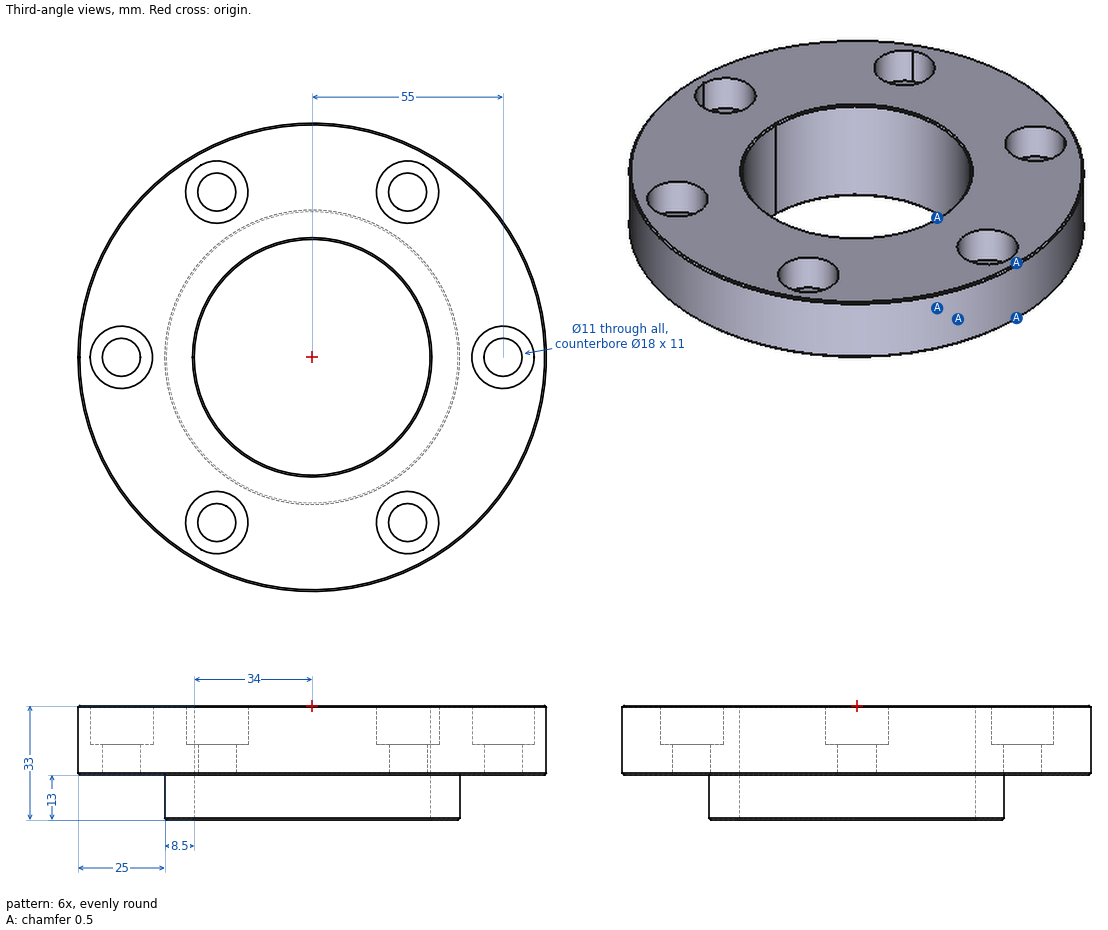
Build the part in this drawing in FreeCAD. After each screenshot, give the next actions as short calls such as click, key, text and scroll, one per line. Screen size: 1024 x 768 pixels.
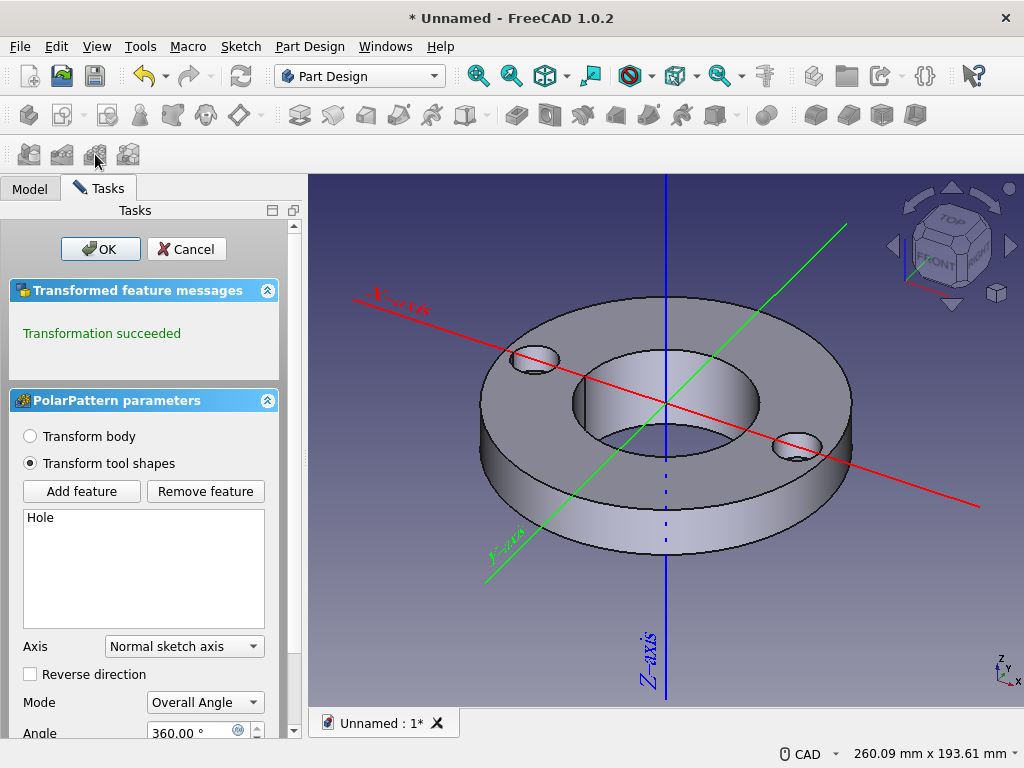
click(185, 646)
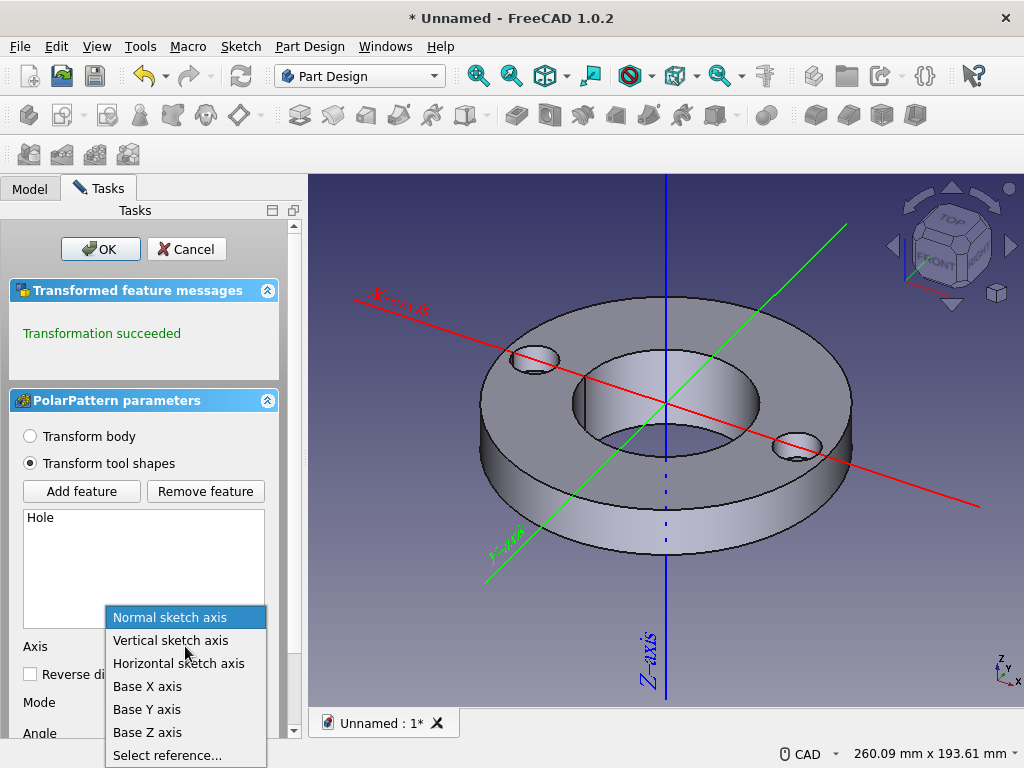
click(184, 732)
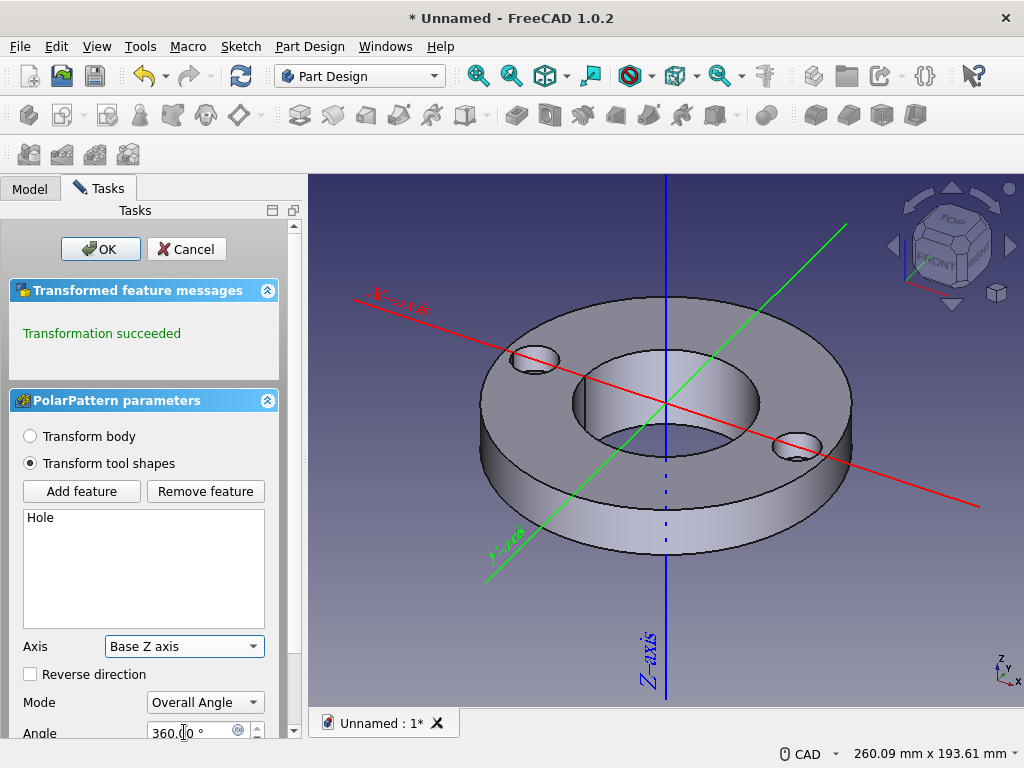
scroll(294, 479, down, 2)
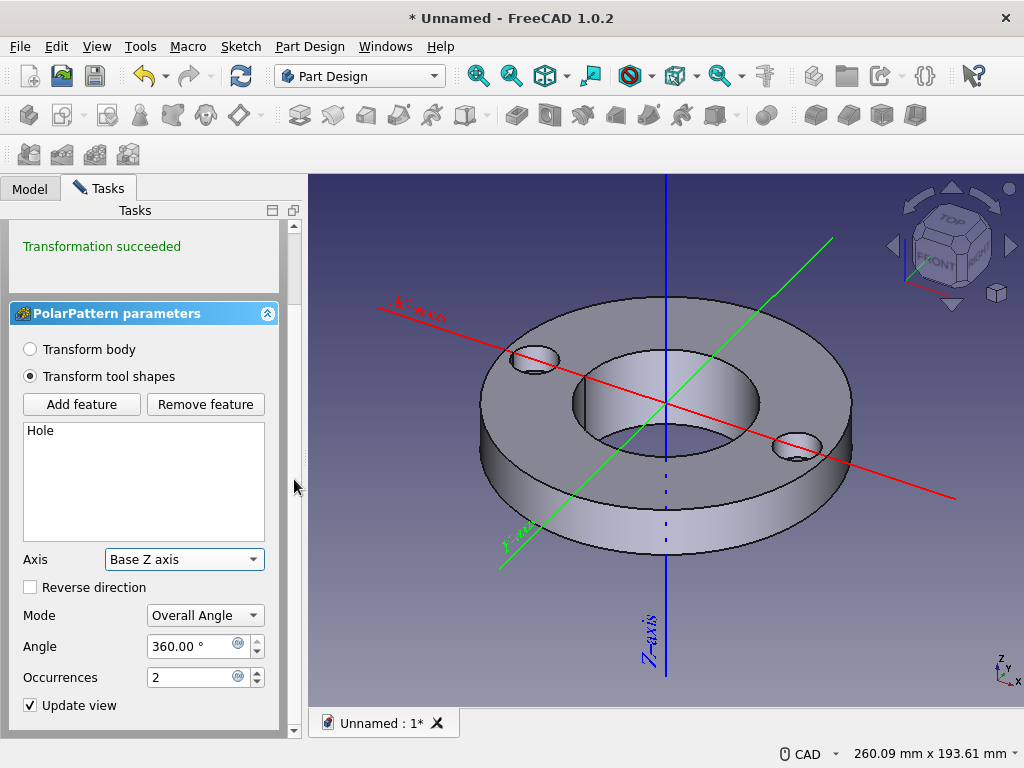
triple_click(199, 678)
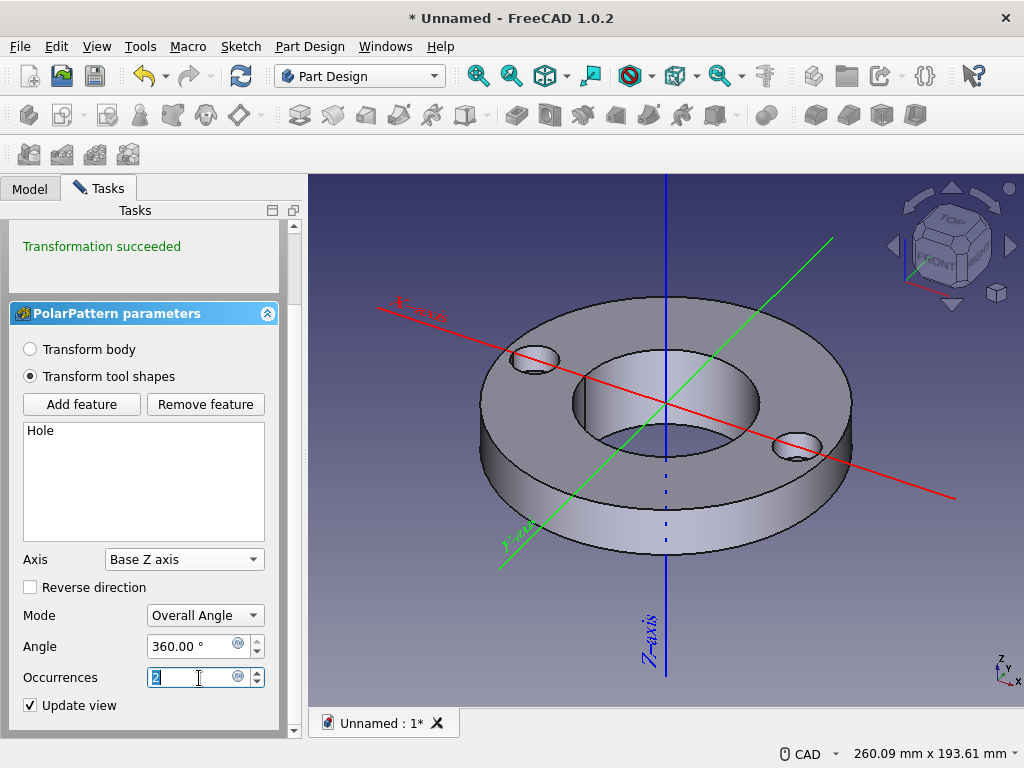
text(6)
key(Tab)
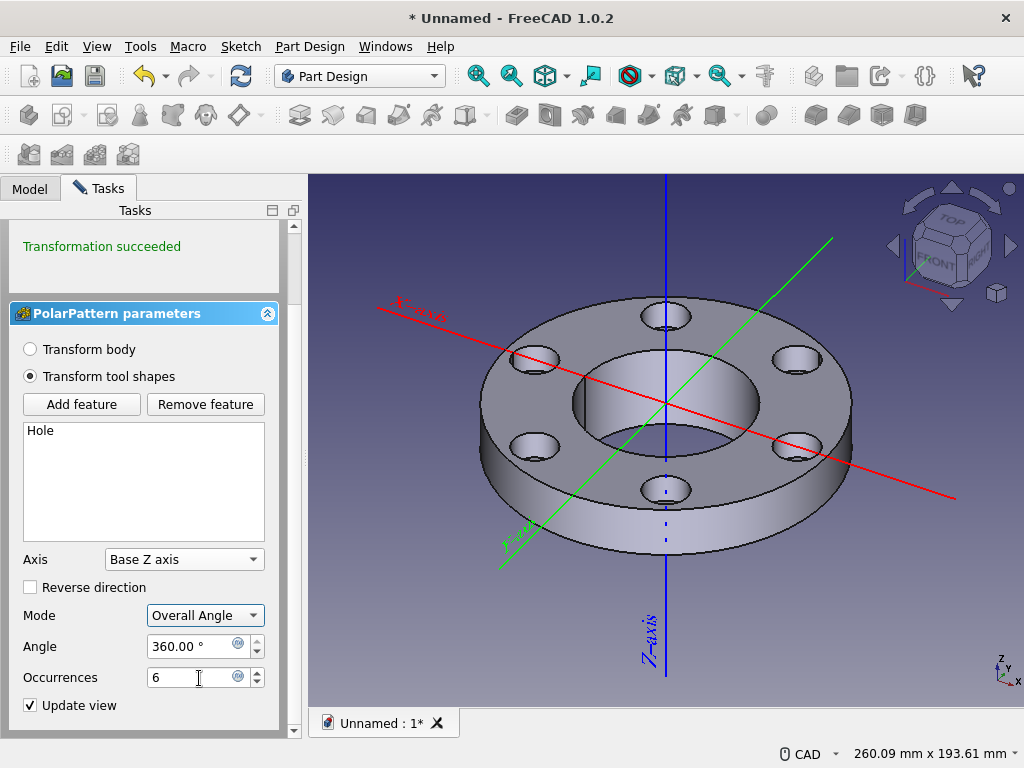
scroll(294, 479, up, 3)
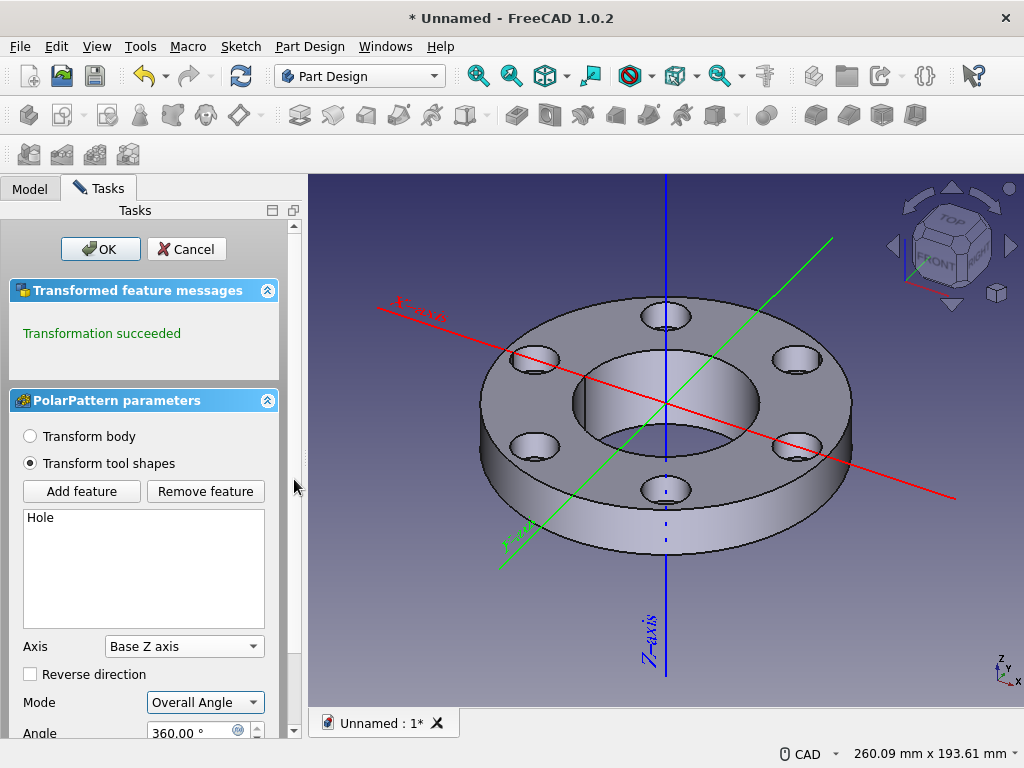
click(101, 249)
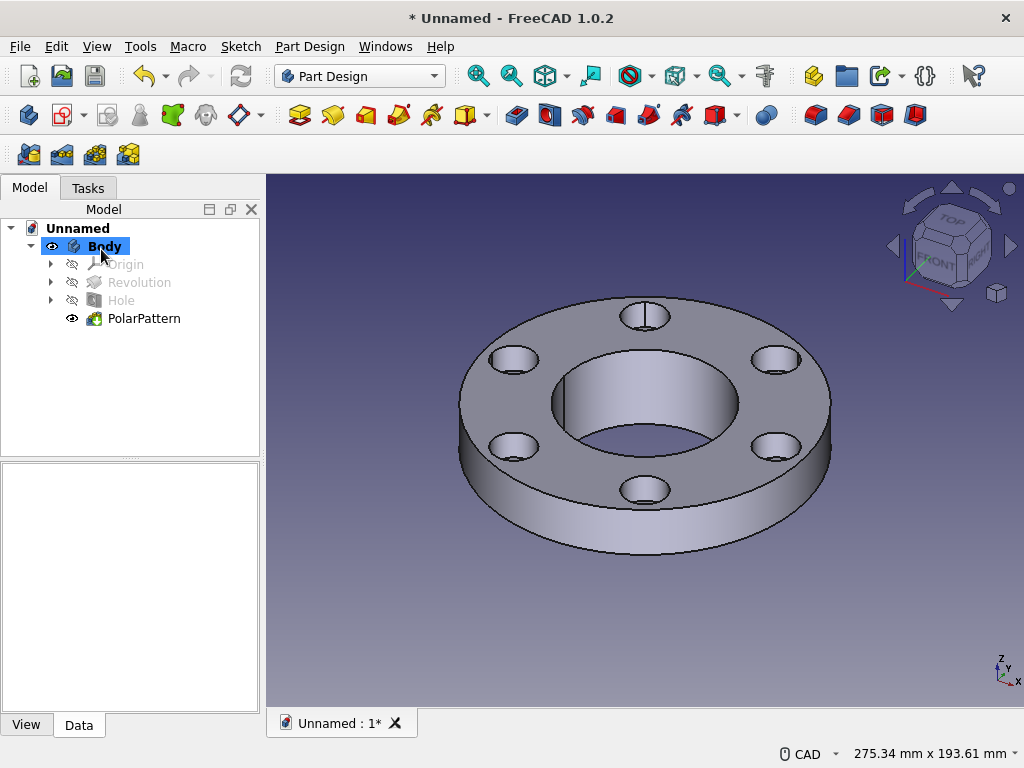
click(806, 456)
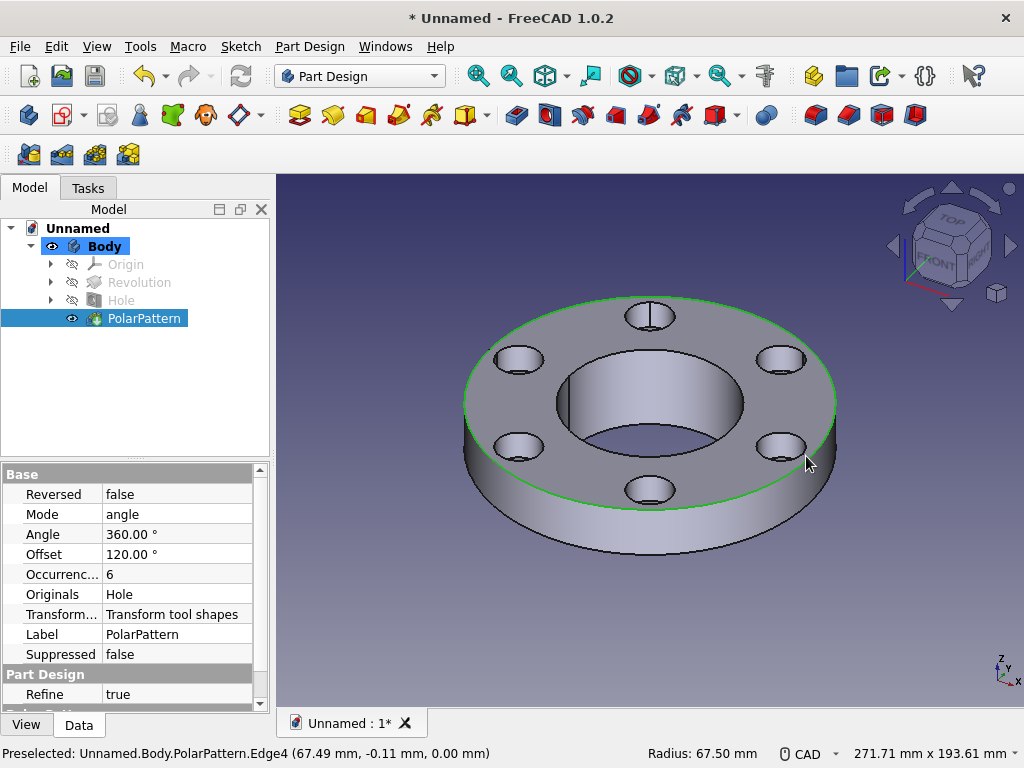
click(743, 397, ctrl)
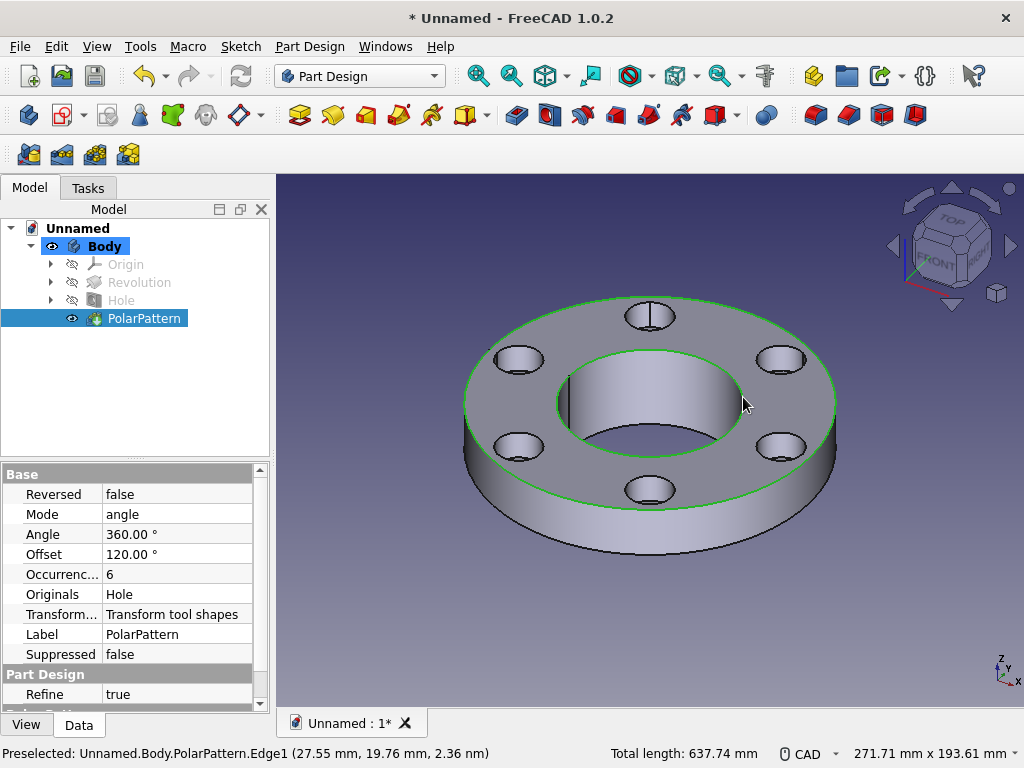
key(0)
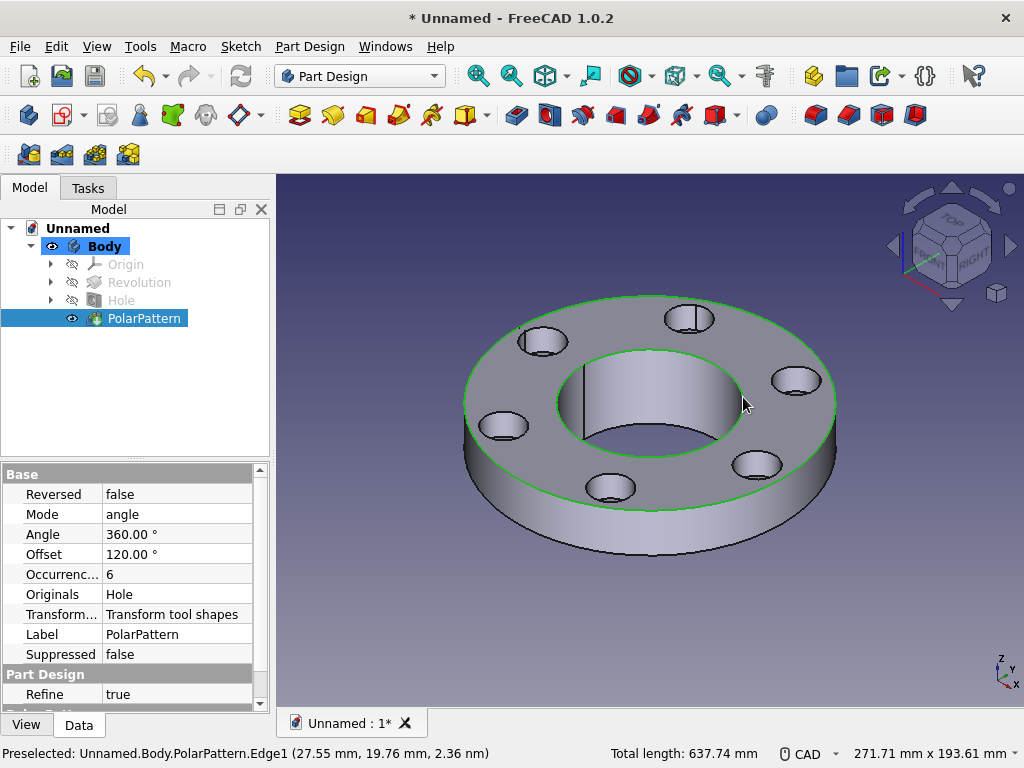
key(2)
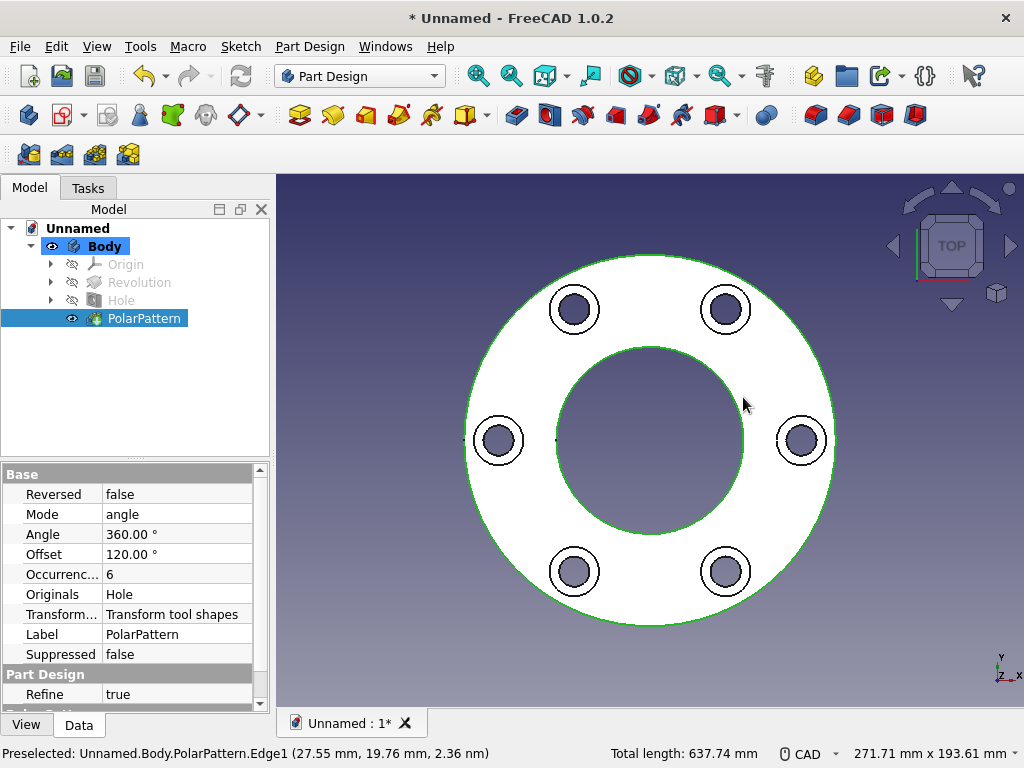
key(1)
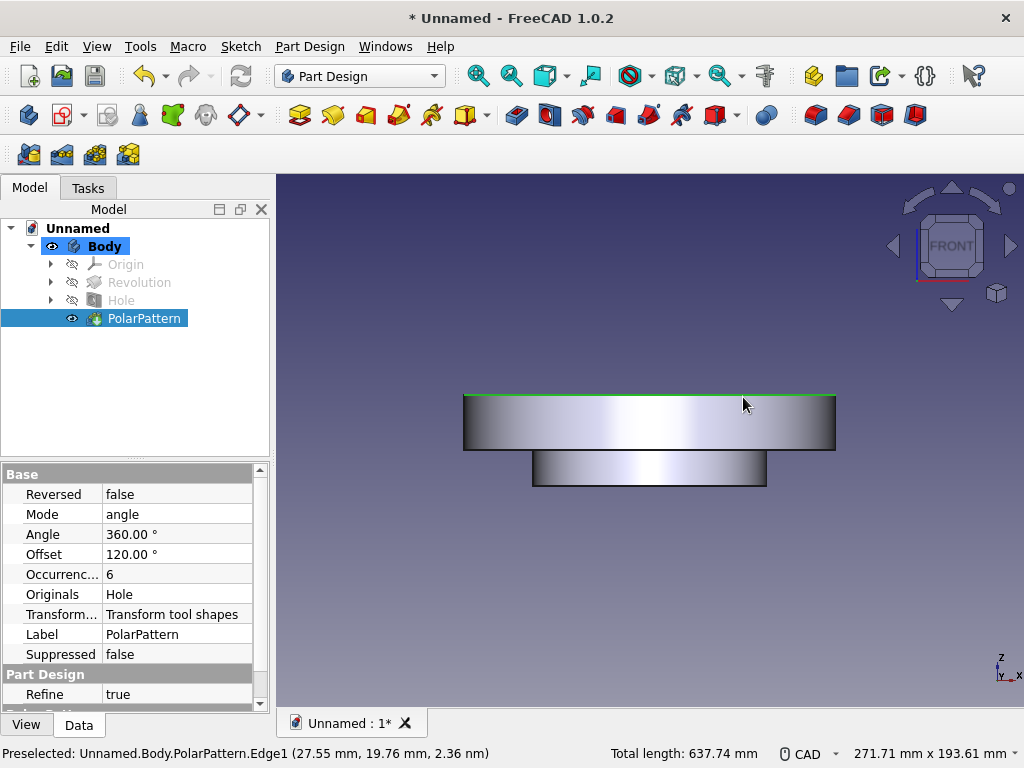
click(535, 485, ctrl)